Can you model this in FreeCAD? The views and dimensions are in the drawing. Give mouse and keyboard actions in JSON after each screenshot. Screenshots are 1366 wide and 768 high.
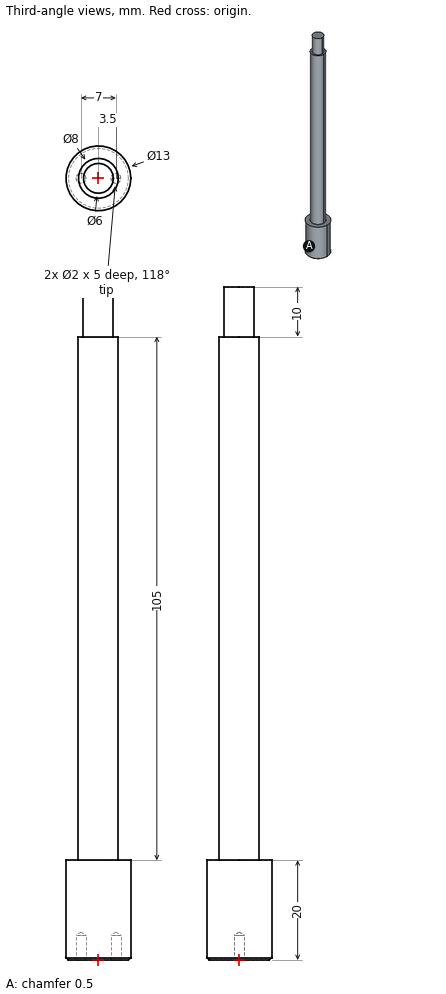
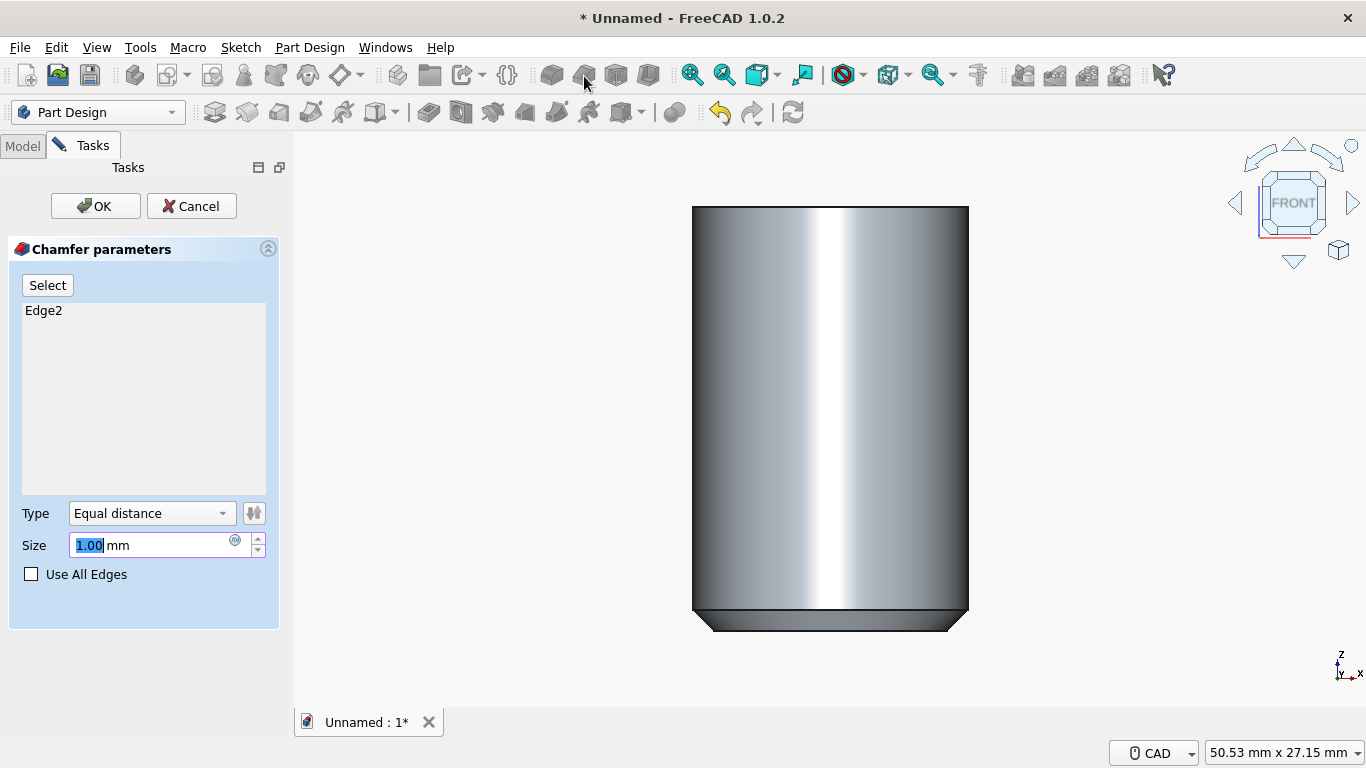
{"action": "type", "text": "0.5"}
{"action": "key", "text": "Tab"}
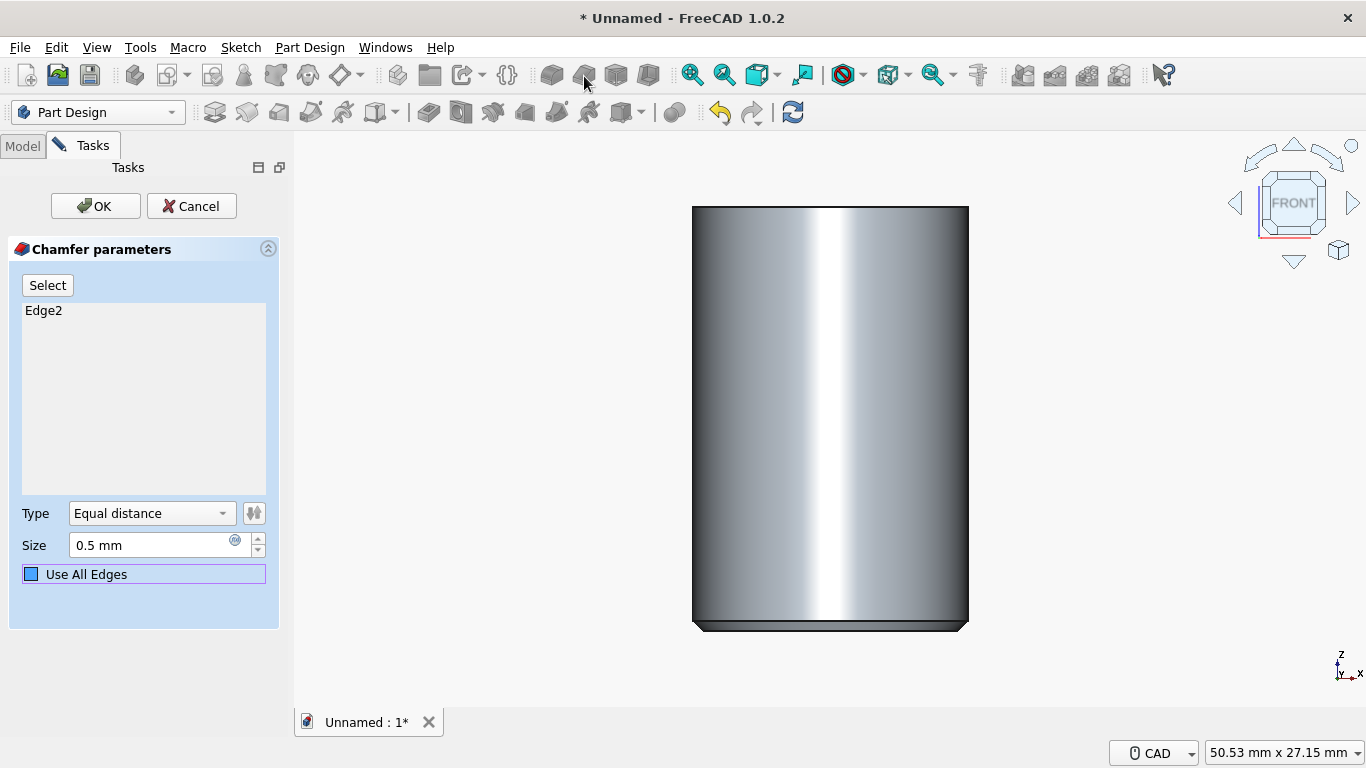
{"action": "left_click", "coordinate": [96, 206]}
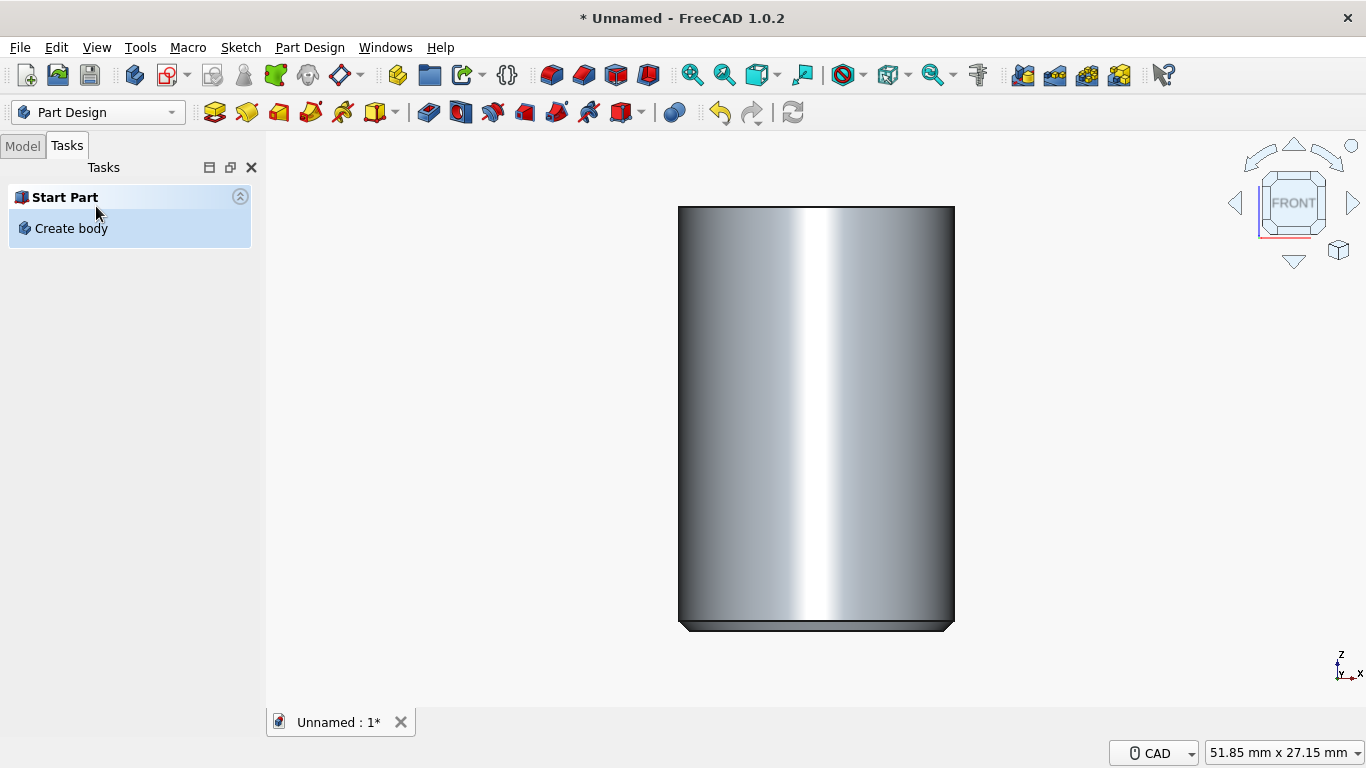
{"action": "key", "text": "5"}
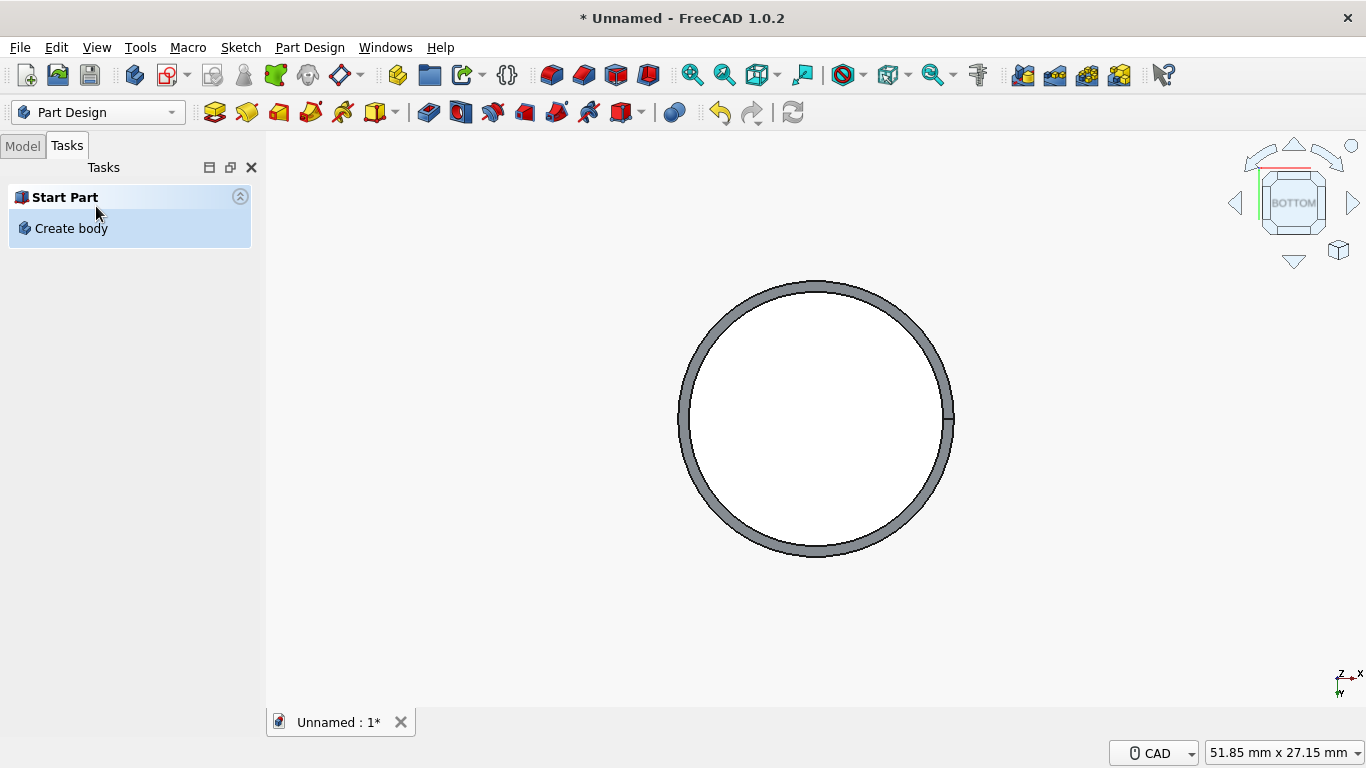
{"action": "left_click", "coordinate": [816, 418]}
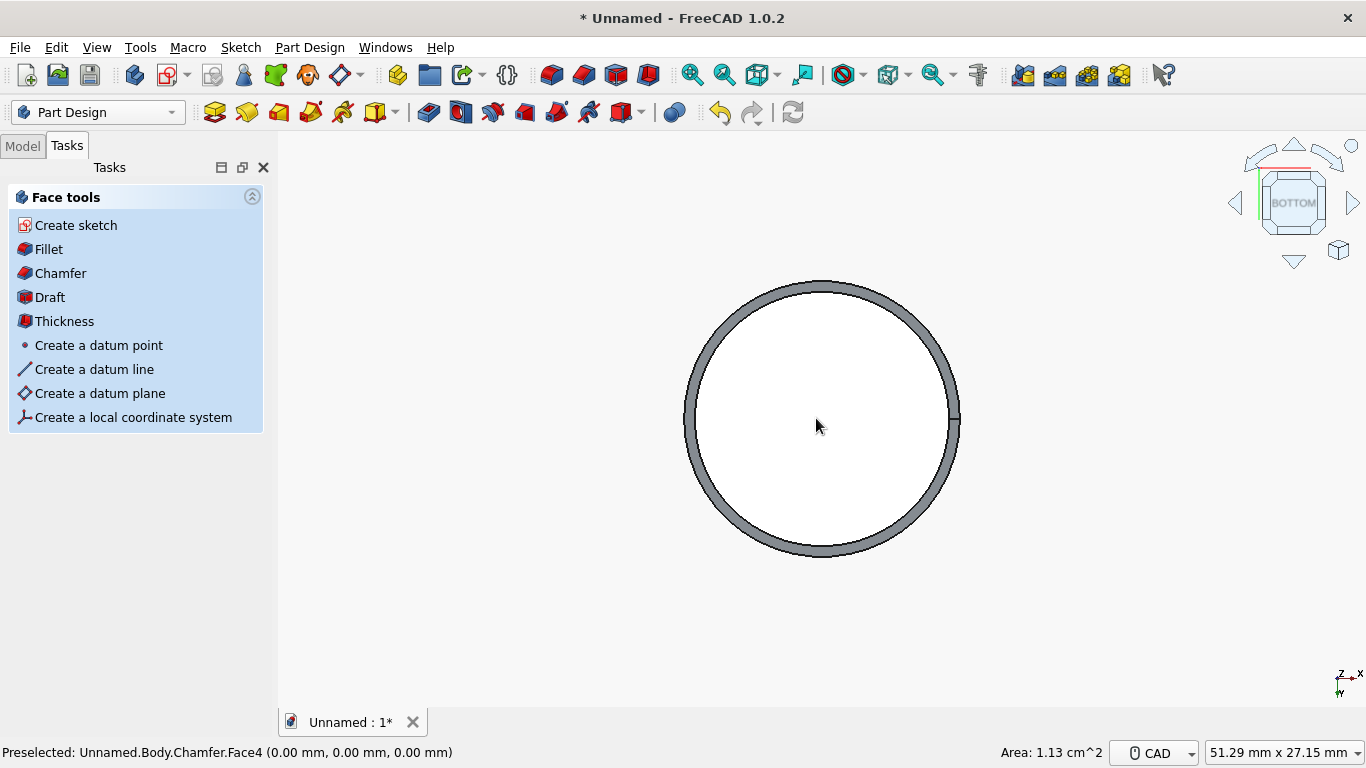
{"action": "left_click", "coordinate": [168, 76]}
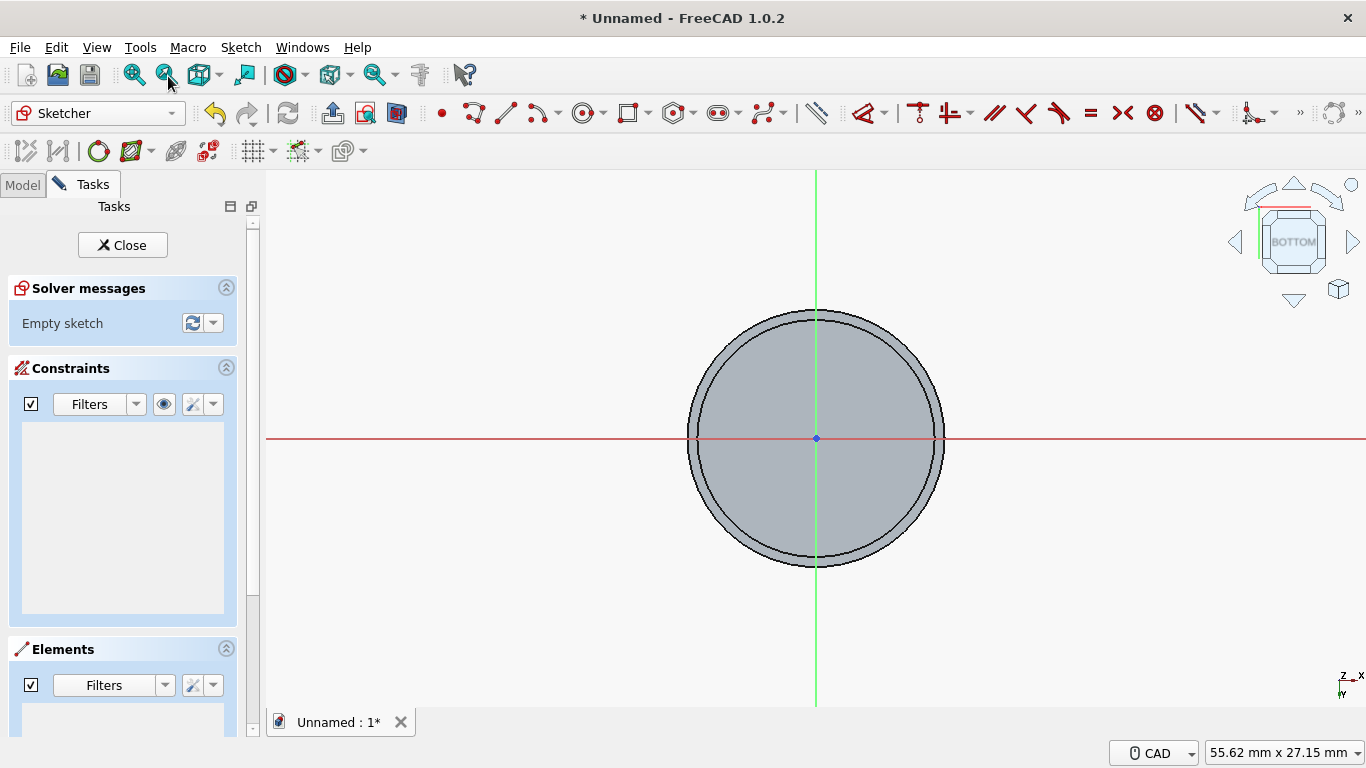
{"action": "scroll", "coordinate": [846, 438], "scroll_direction": "up", "scroll_amount": 6}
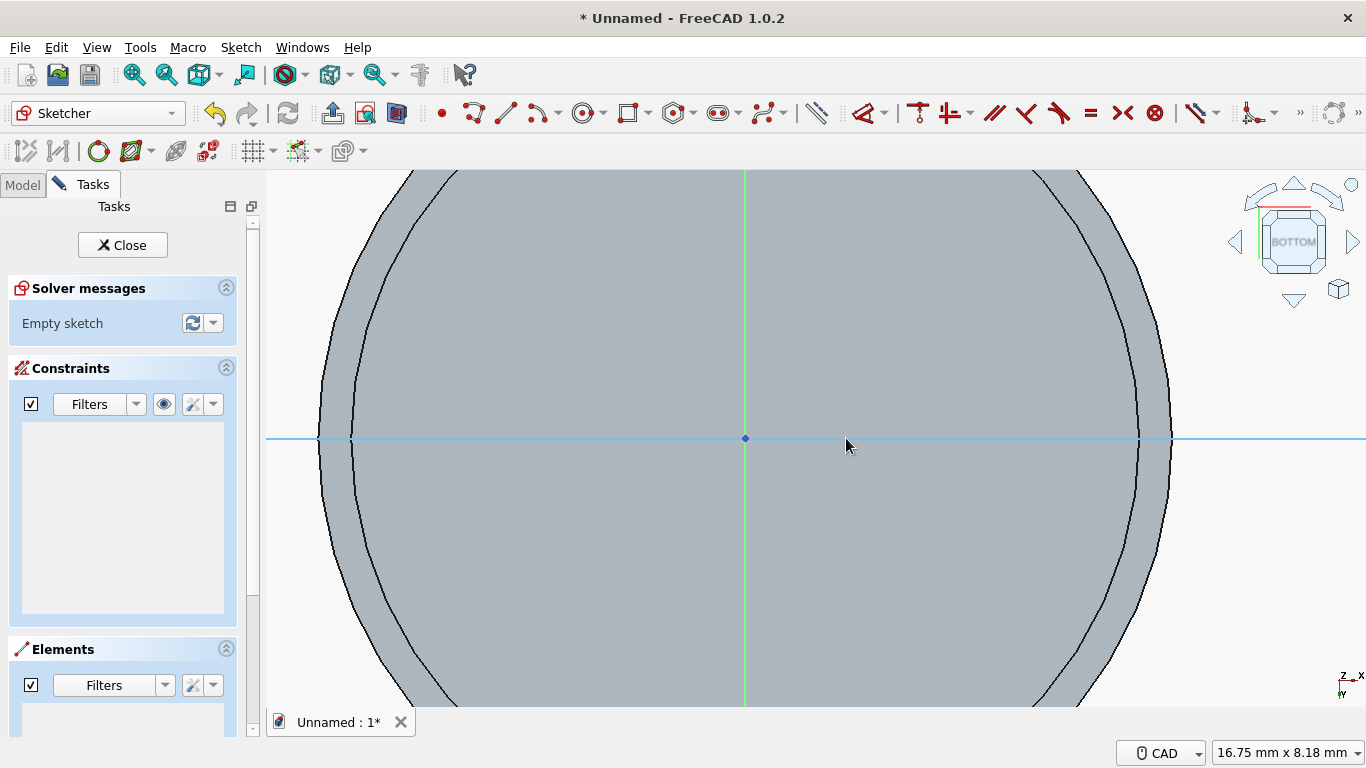
{"action": "key", "text": "g c"}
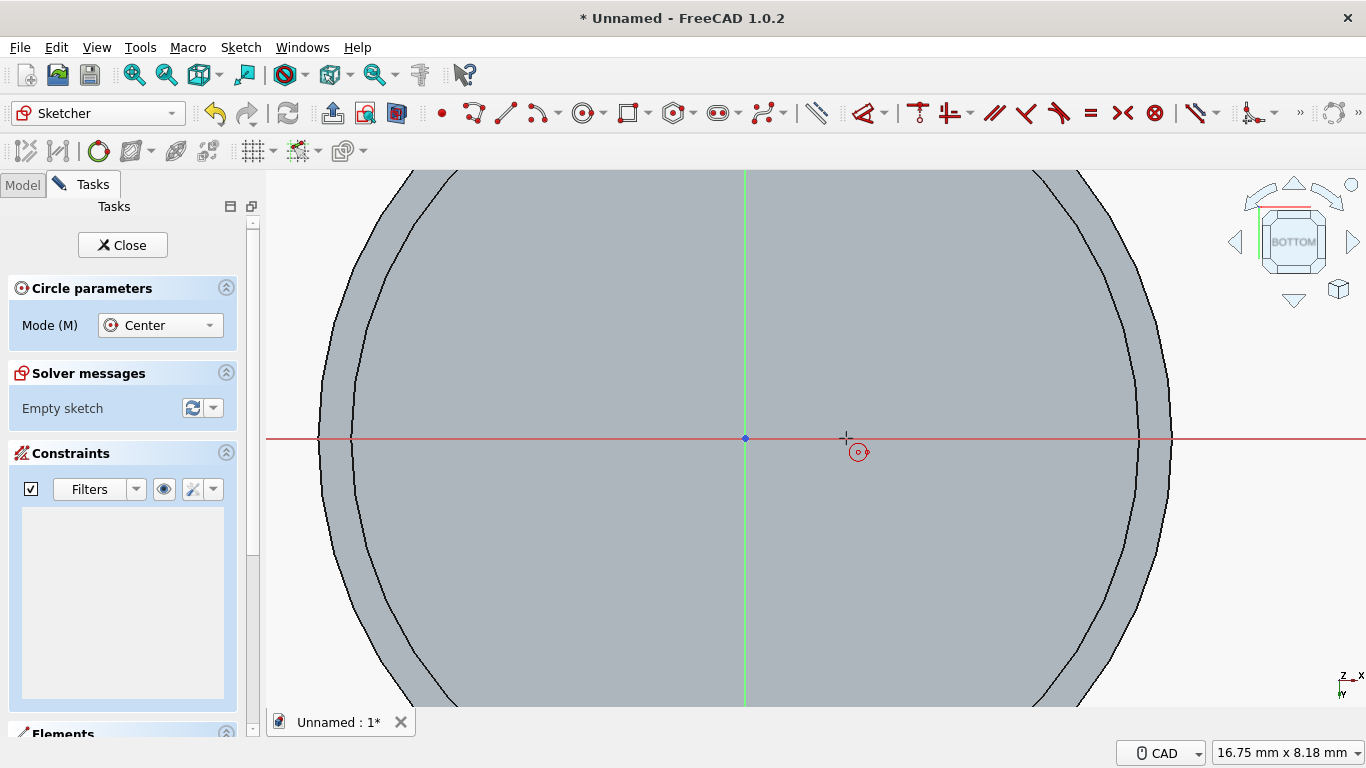
{"action": "left_click", "coordinate": [975, 438]}
{"action": "left_click", "coordinate": [1021, 392]}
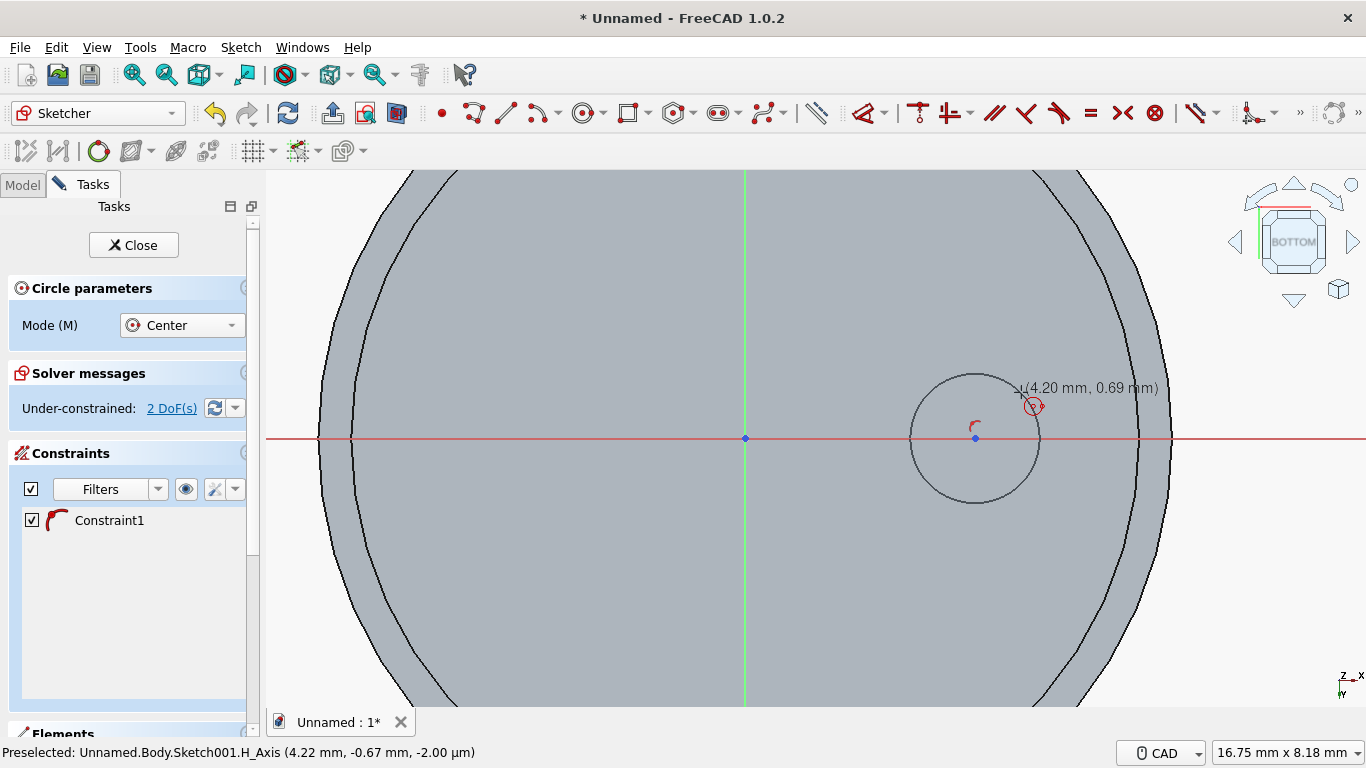
{"action": "left_click", "coordinate": [515, 438]}
{"action": "left_click", "coordinate": [562, 392]}
{"action": "key", "text": "Escape"}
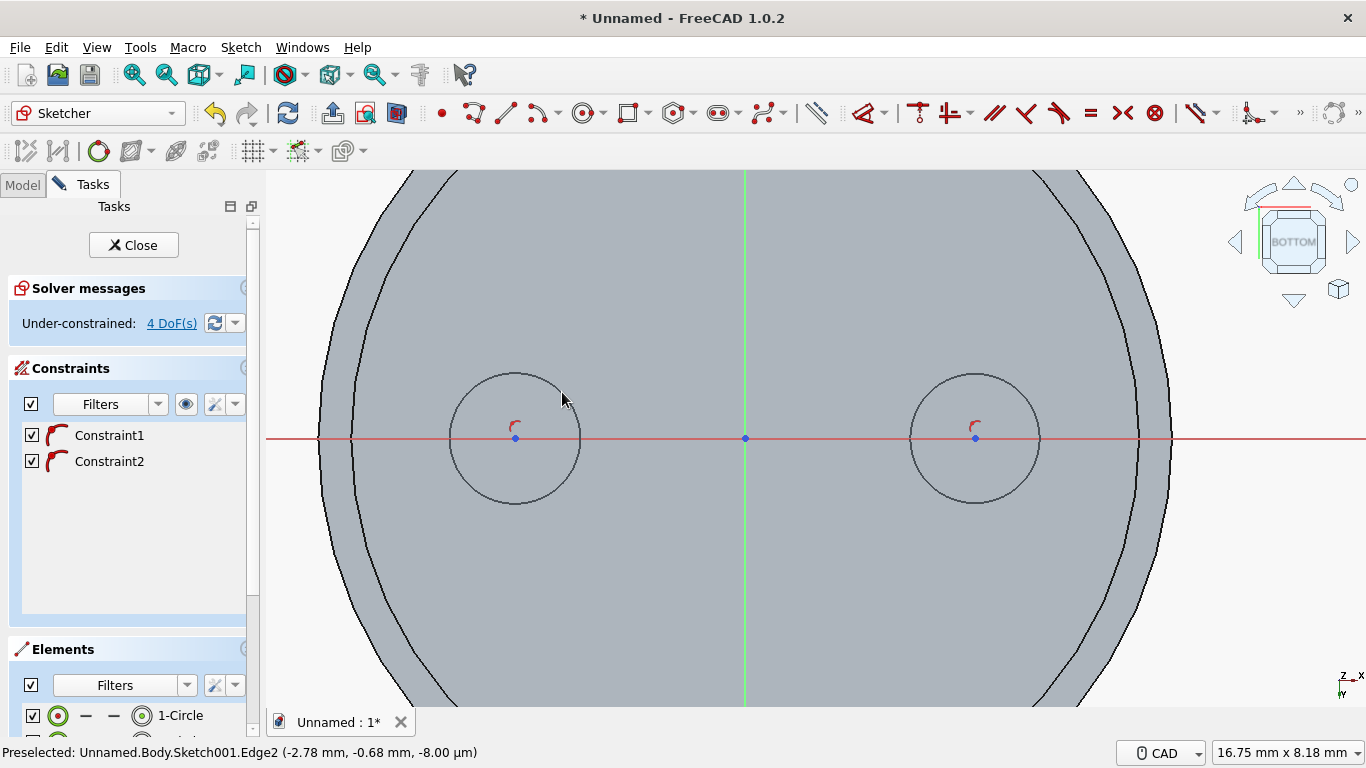
{"action": "left_click", "coordinate": [1021, 393]}